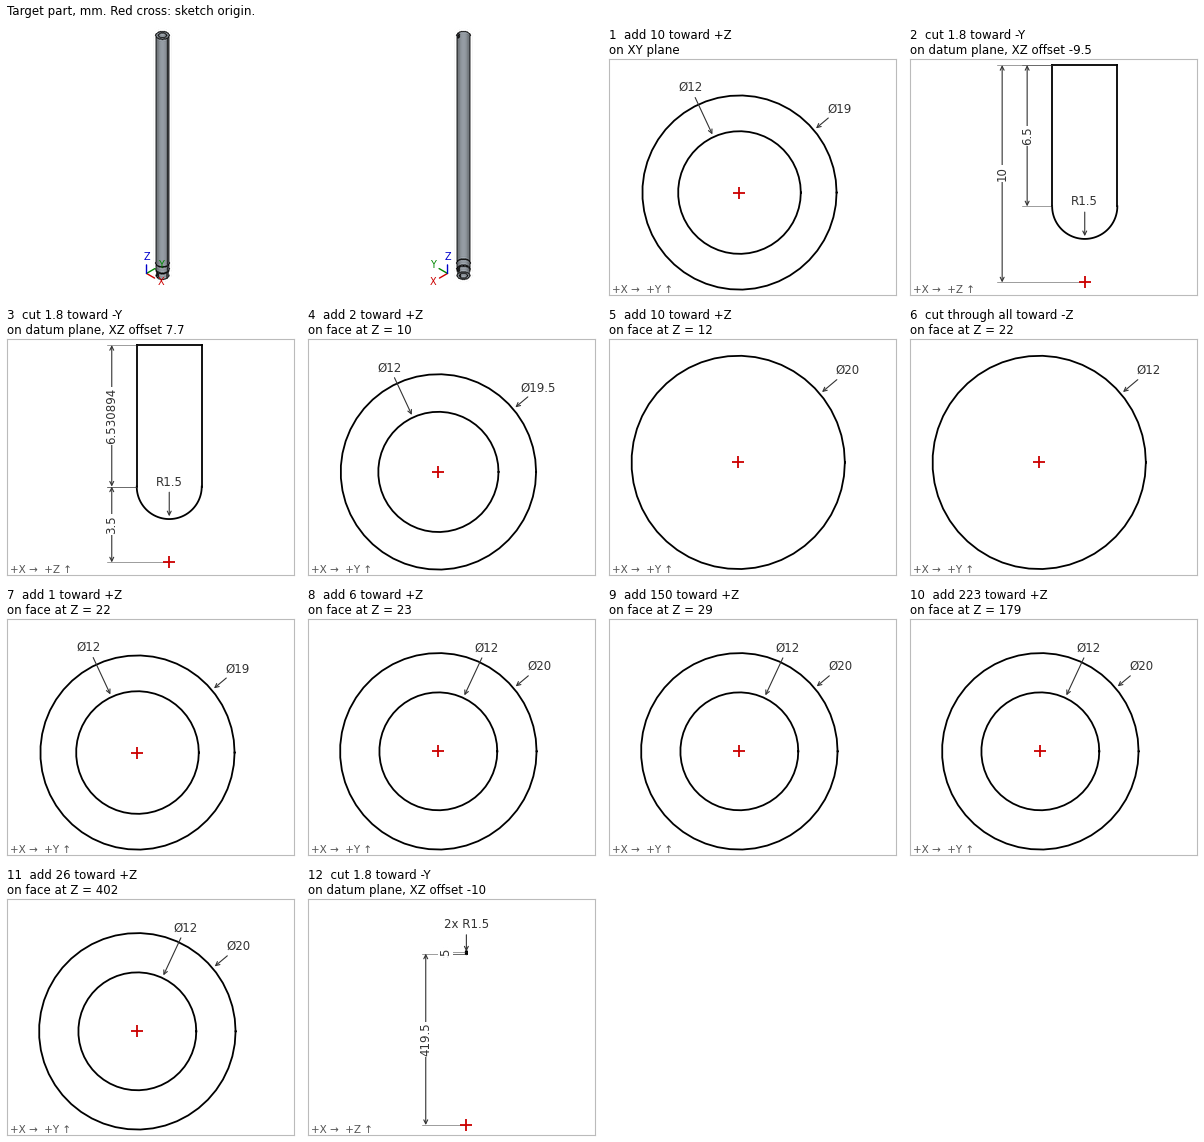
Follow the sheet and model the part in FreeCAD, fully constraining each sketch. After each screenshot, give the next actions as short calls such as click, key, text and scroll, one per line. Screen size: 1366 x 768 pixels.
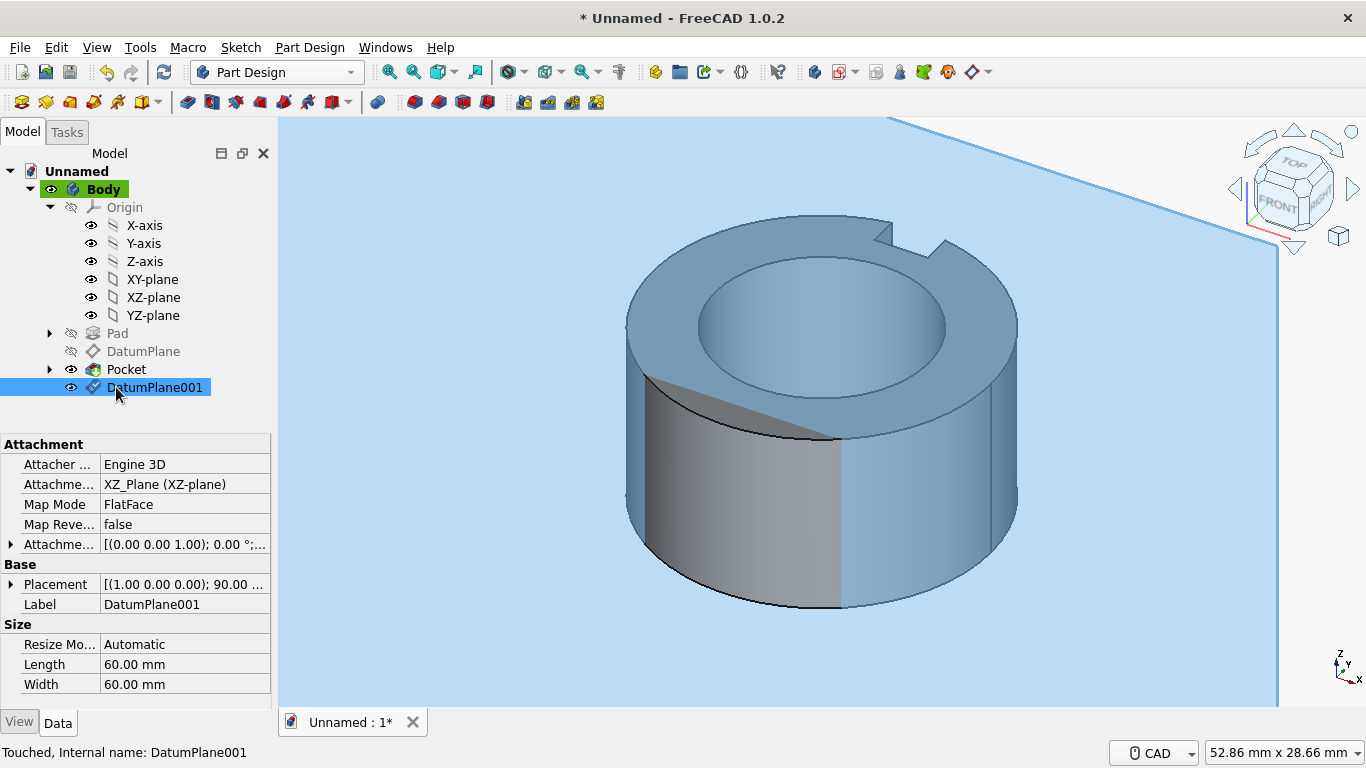
click(840, 72)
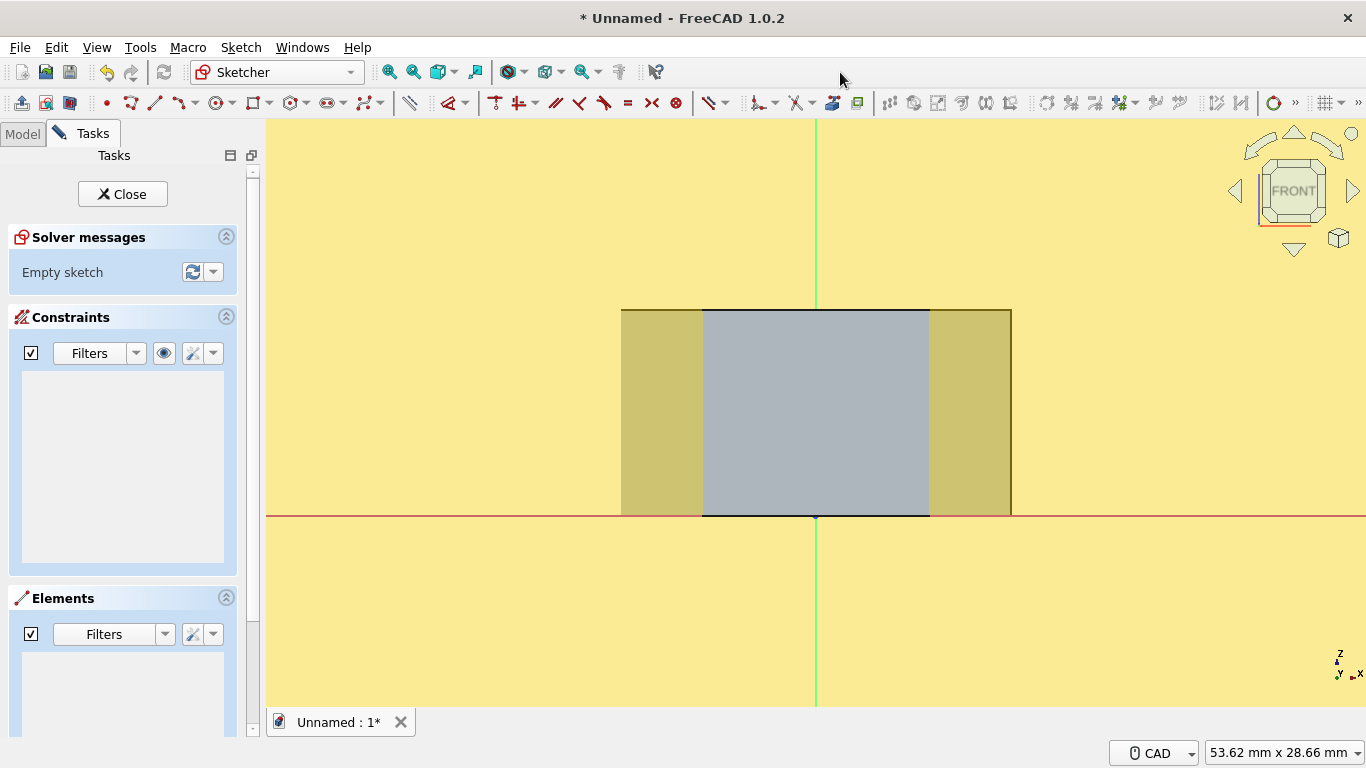
click(70, 104)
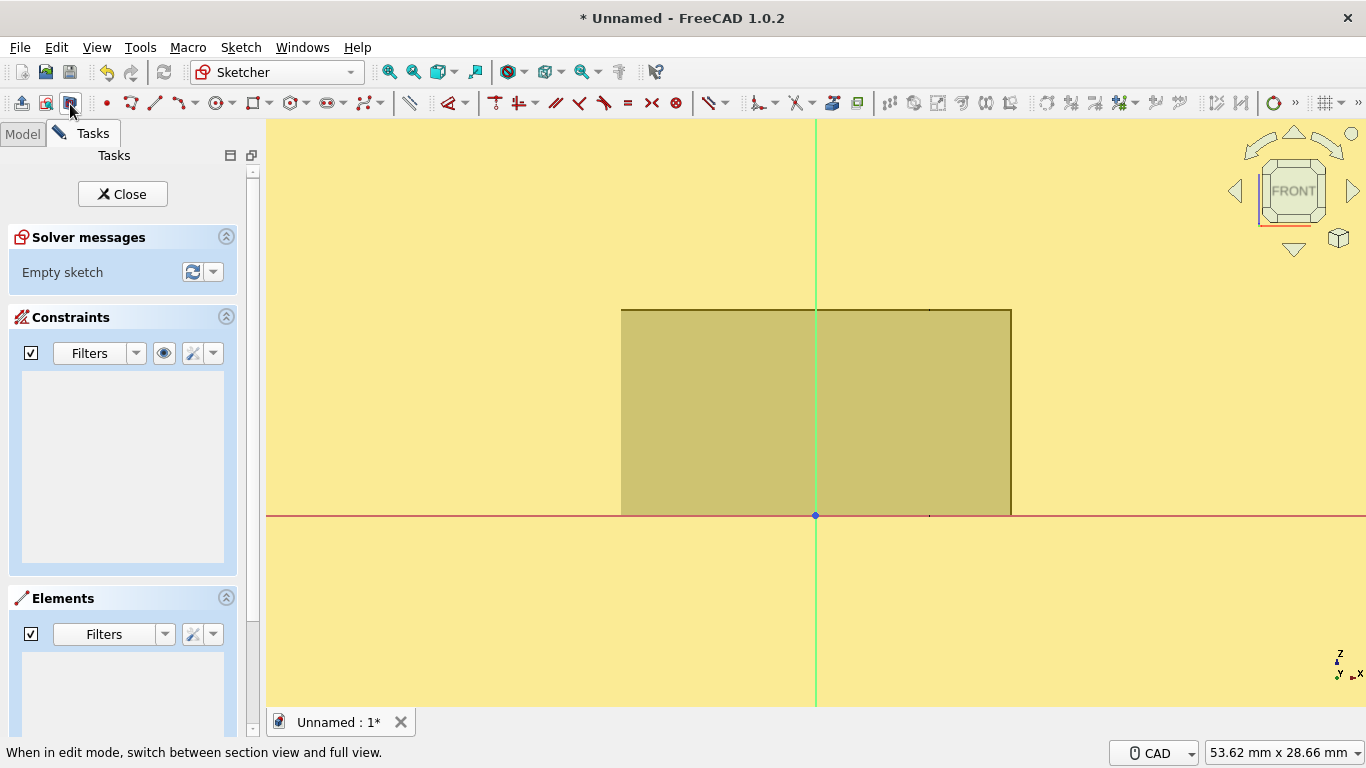
scroll(899, 412, up, 3)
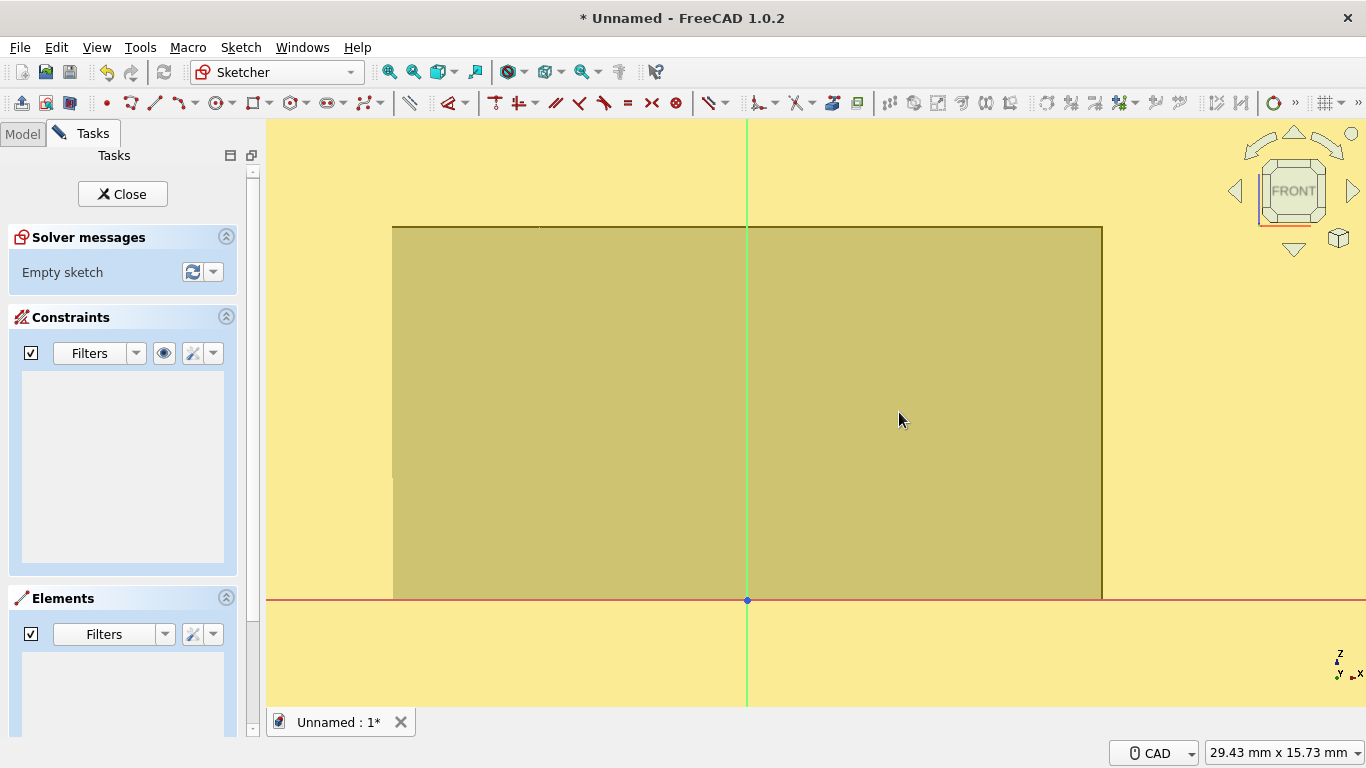
click(132, 104)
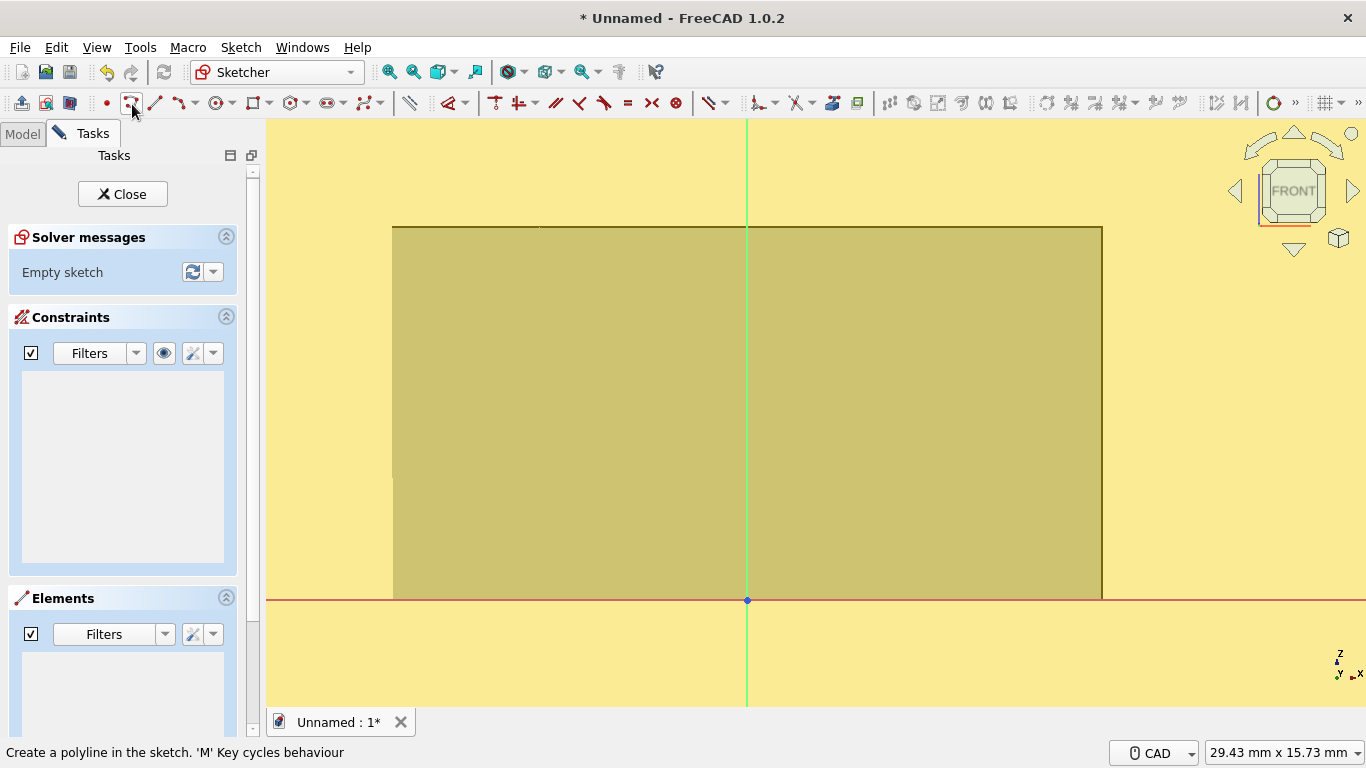
click(691, 469)
click(691, 225)
click(803, 225)
click(803, 469)
right_click(803, 469)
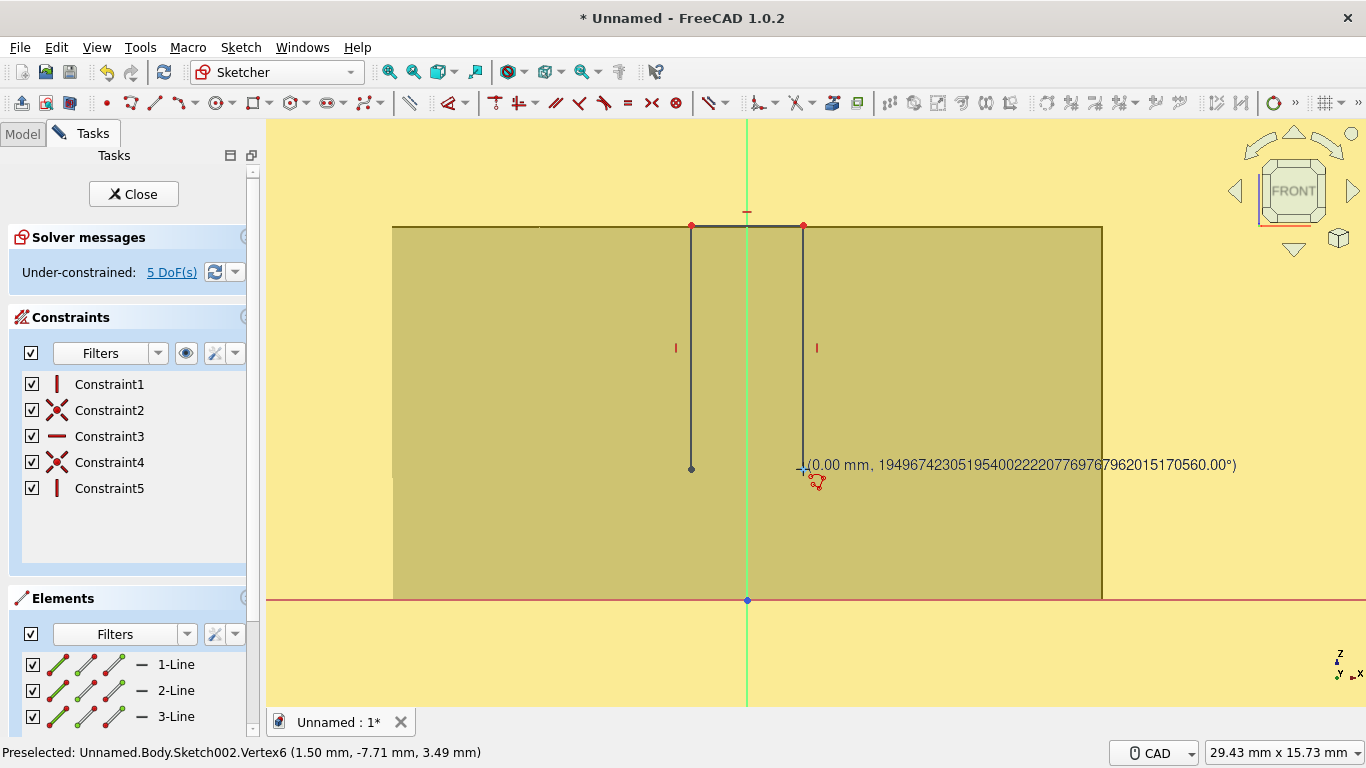
click(180, 104)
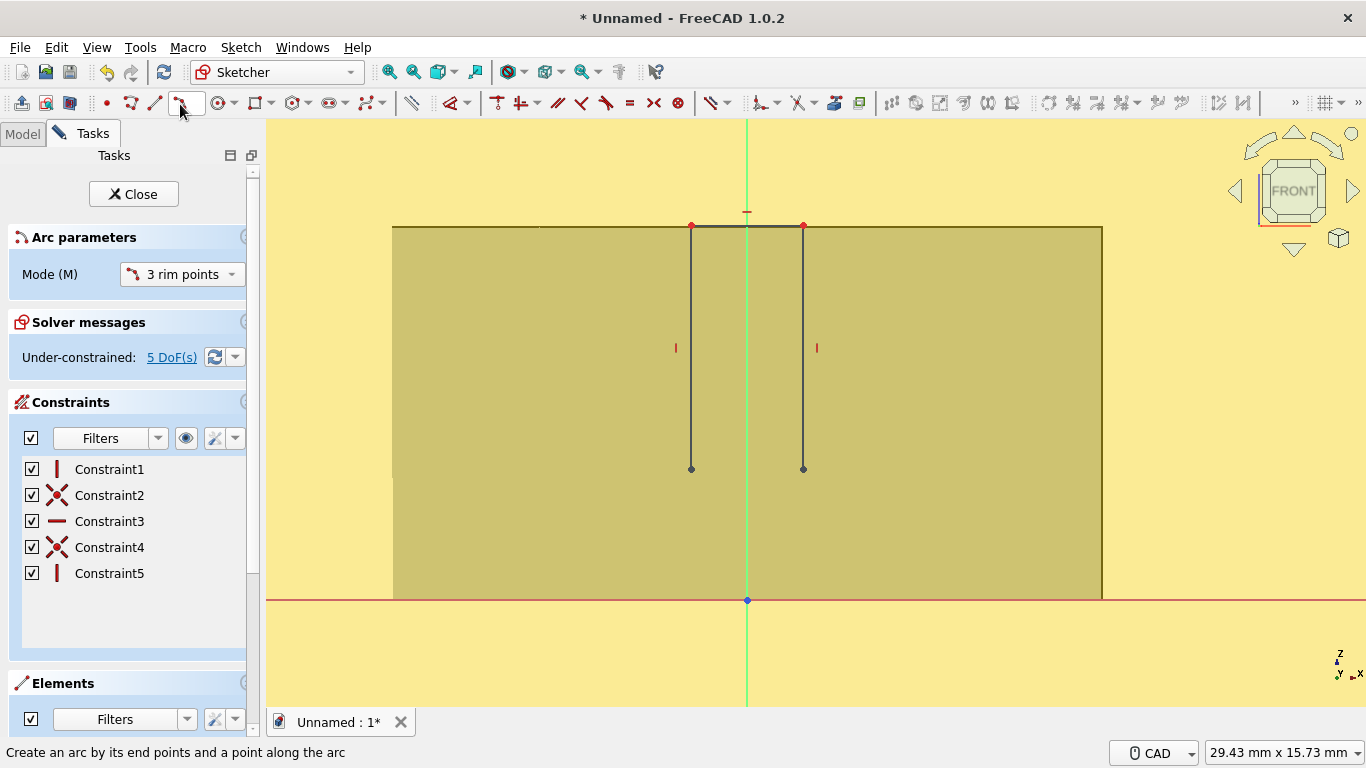
click(803, 470)
click(691, 470)
click(730, 523)
key(Escape)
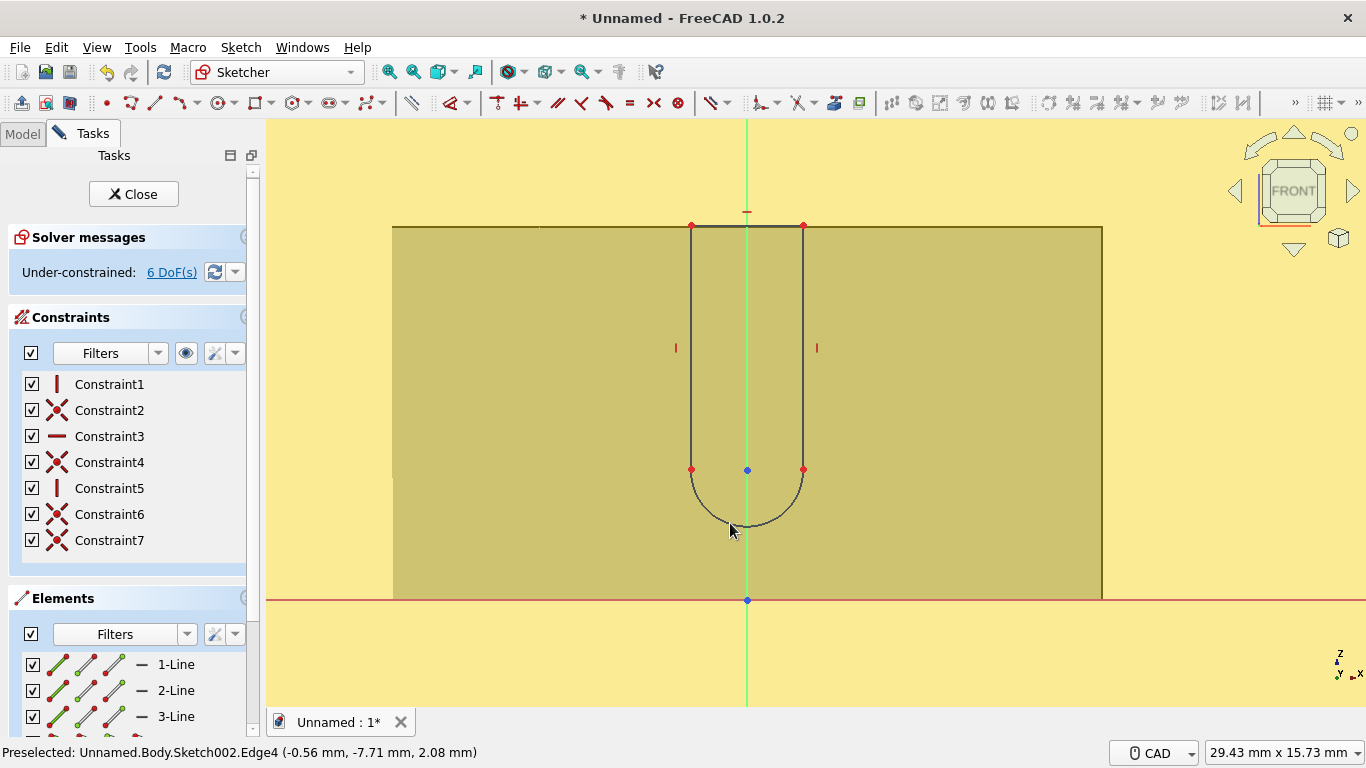
click(691, 397)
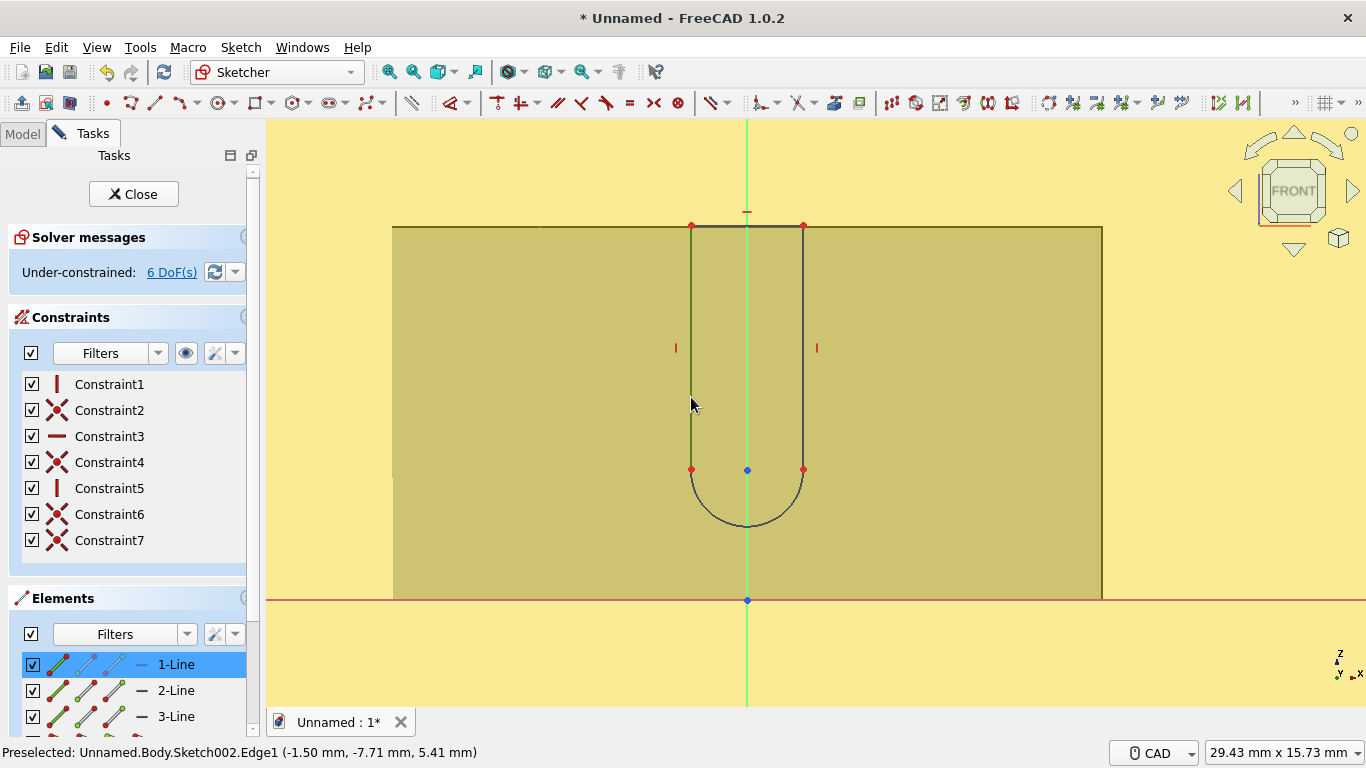
click(714, 516)